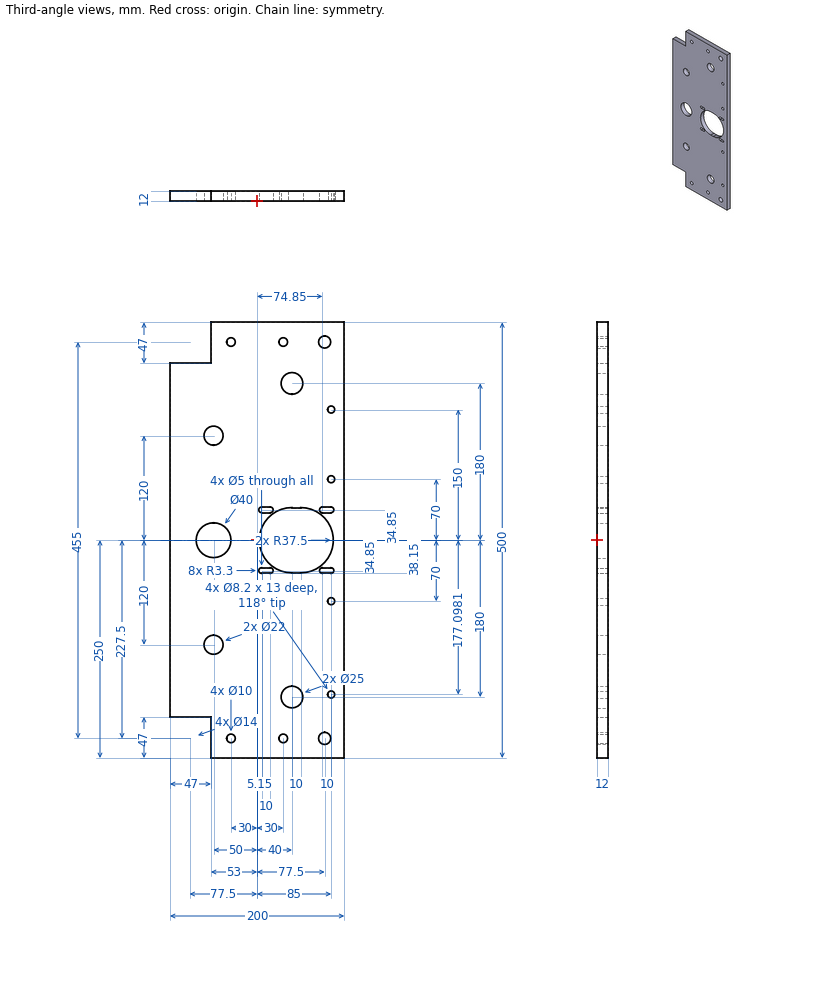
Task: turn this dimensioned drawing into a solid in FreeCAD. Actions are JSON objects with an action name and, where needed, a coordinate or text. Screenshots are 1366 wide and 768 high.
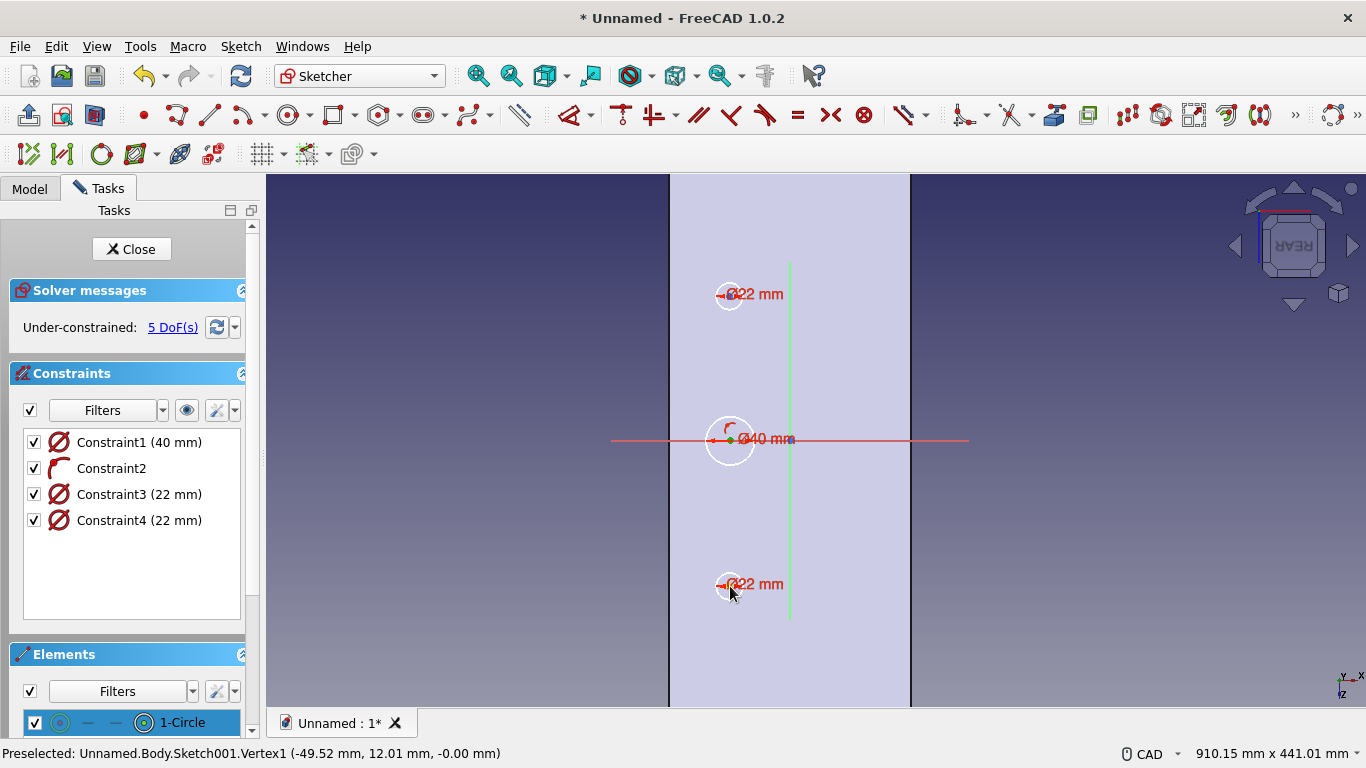
{"action": "left_click", "coordinate": [730, 296]}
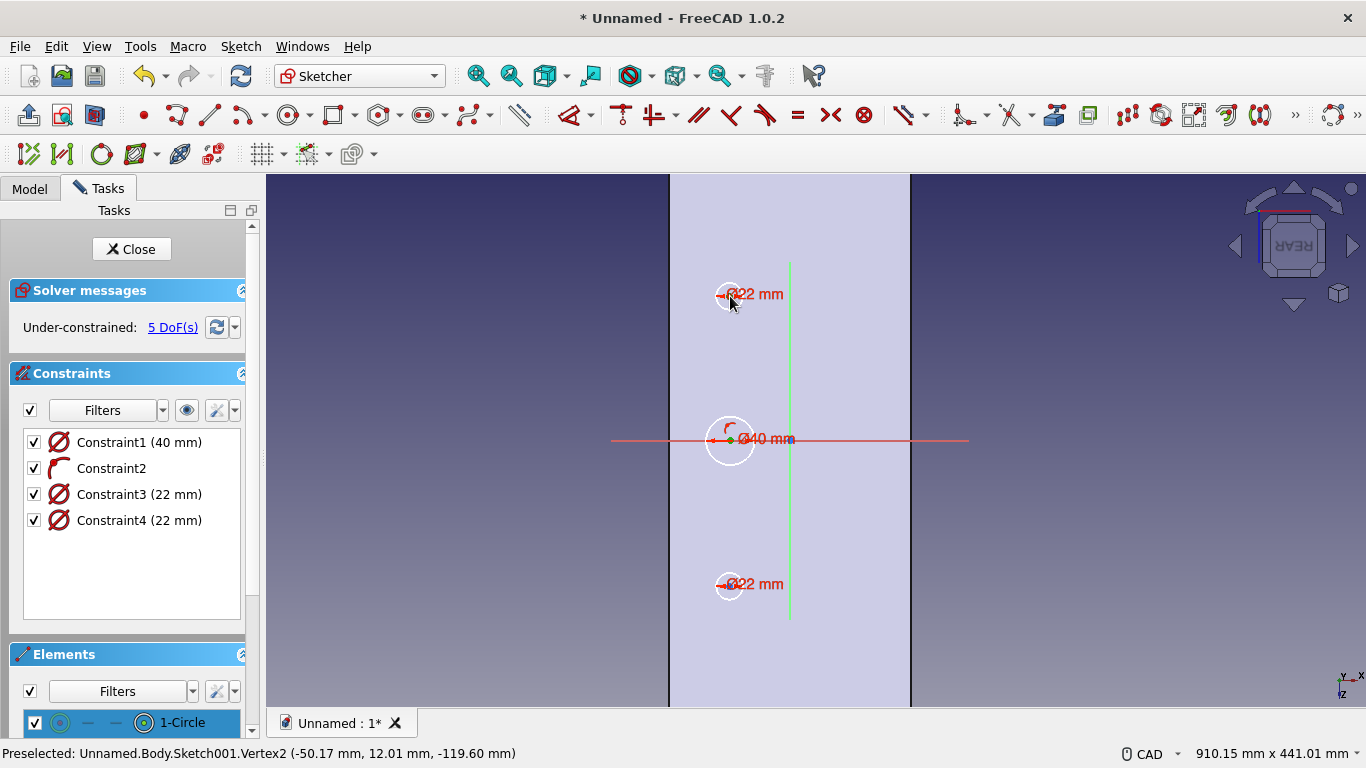
{"action": "key", "text": "v"}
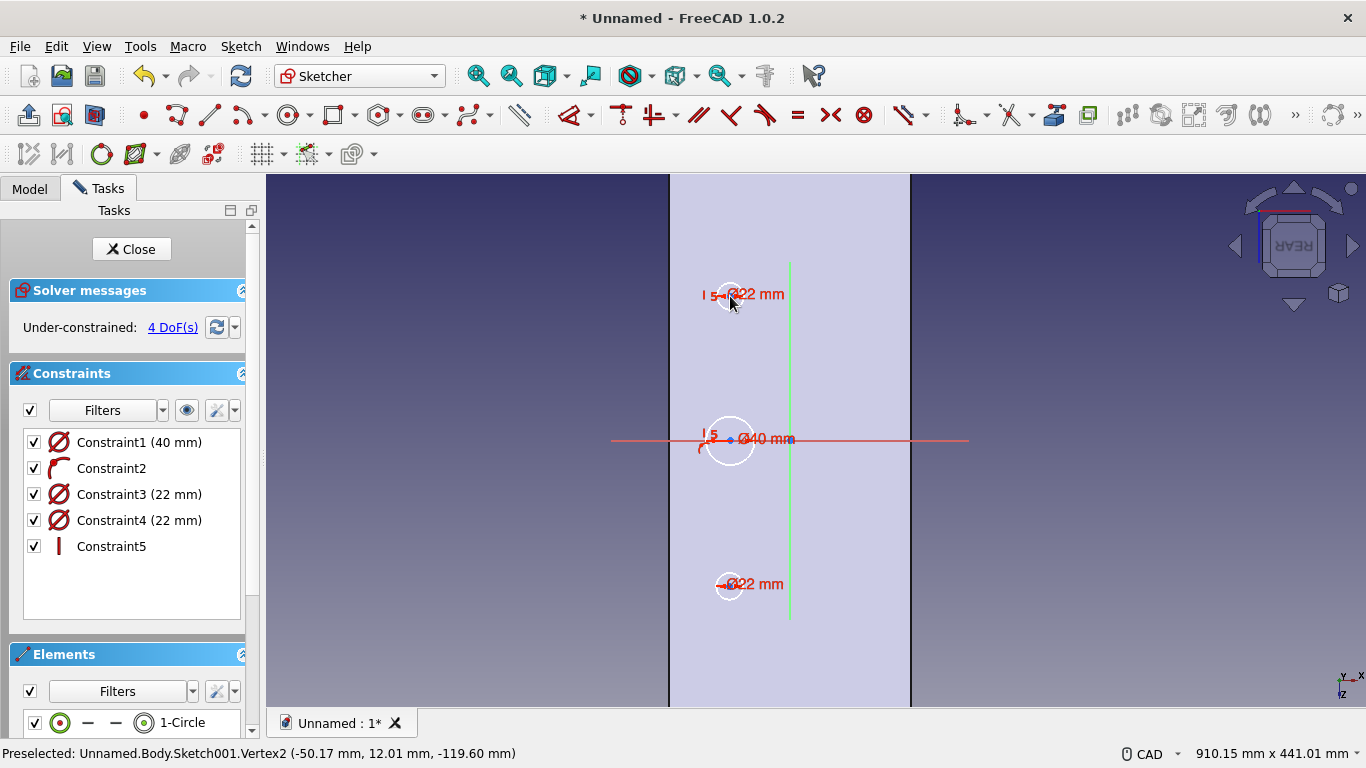
{"action": "left_click", "coordinate": [730, 441]}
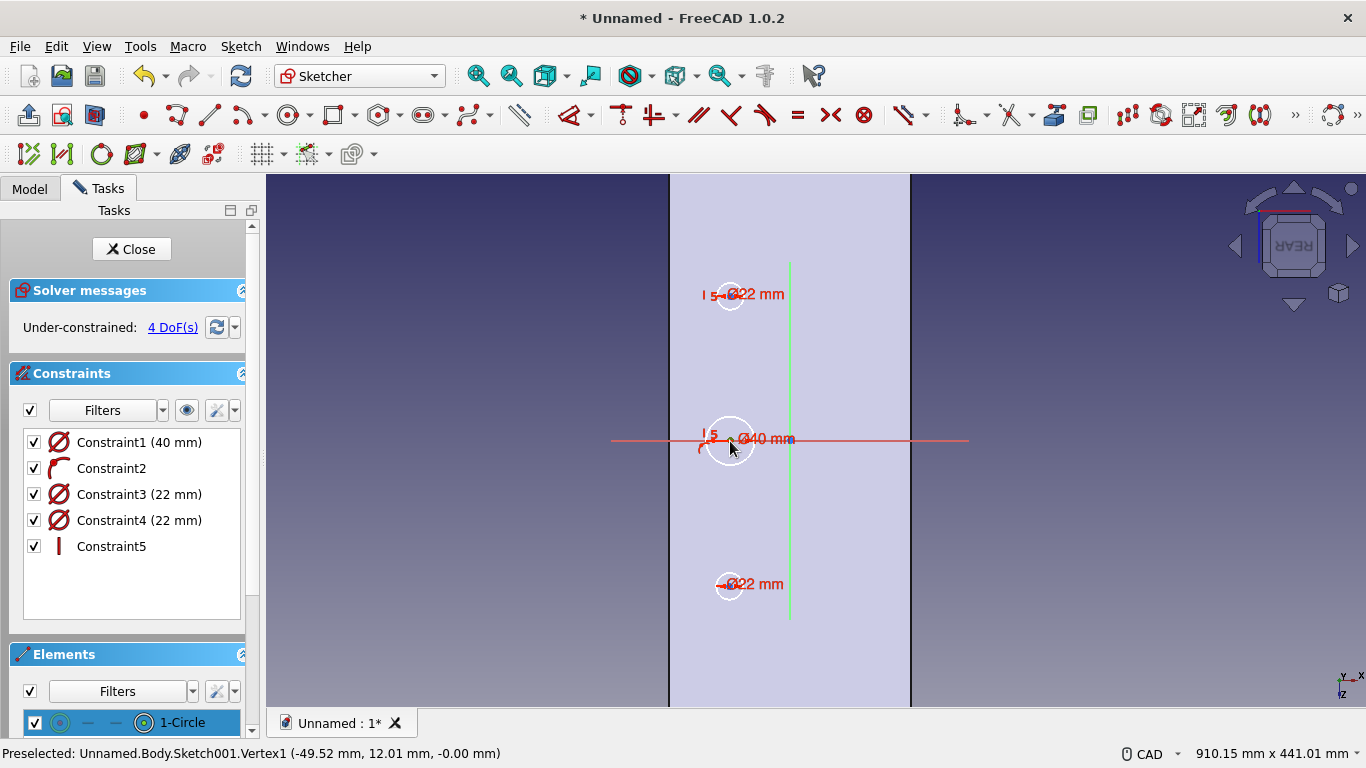
{"action": "left_click", "coordinate": [730, 586]}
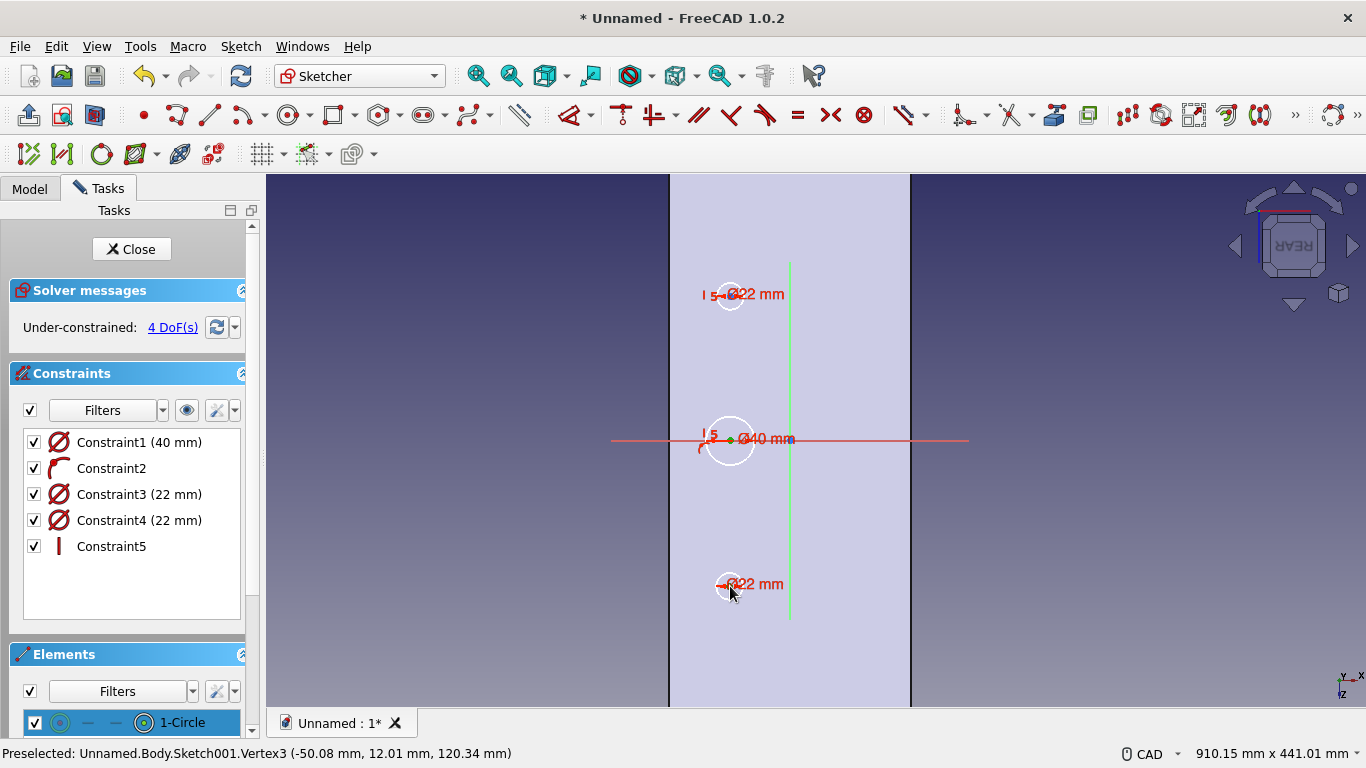
{"action": "key", "text": "v"}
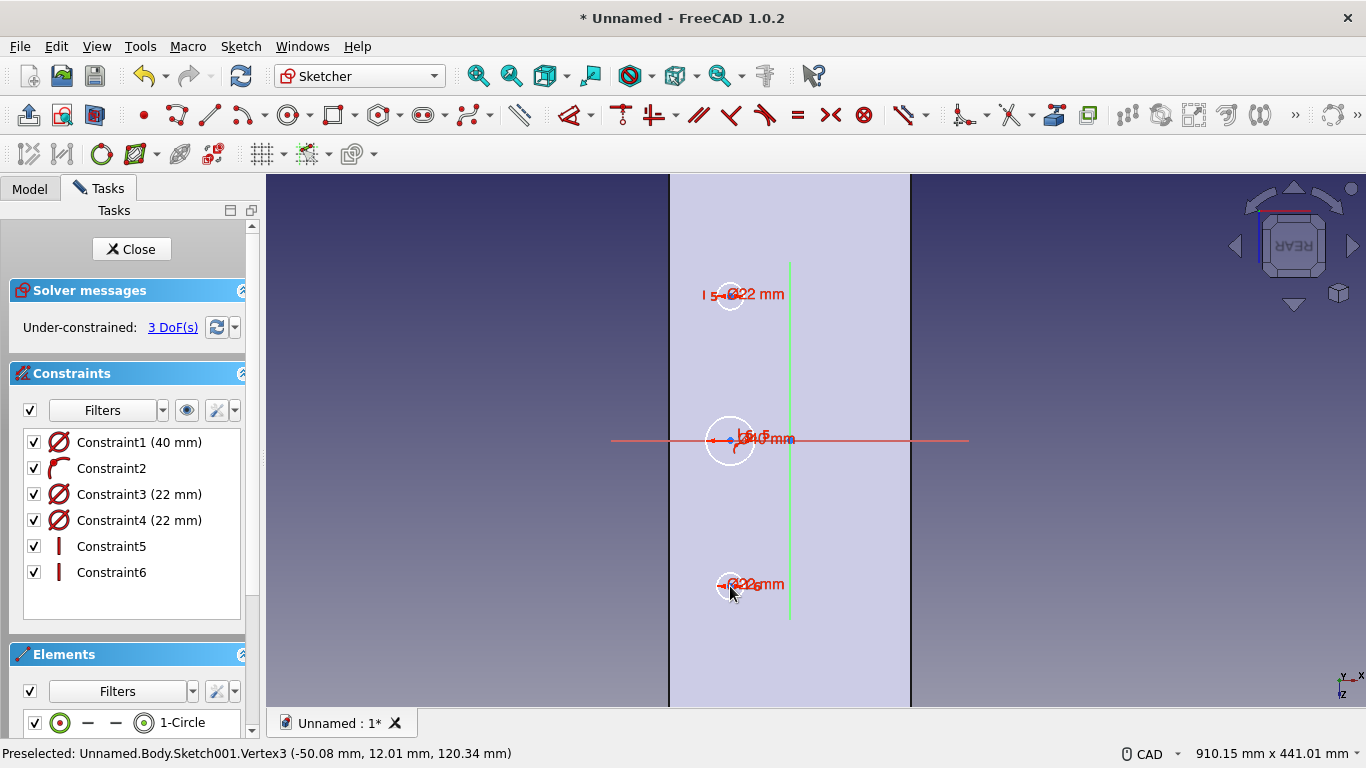
{"action": "key", "text": "d"}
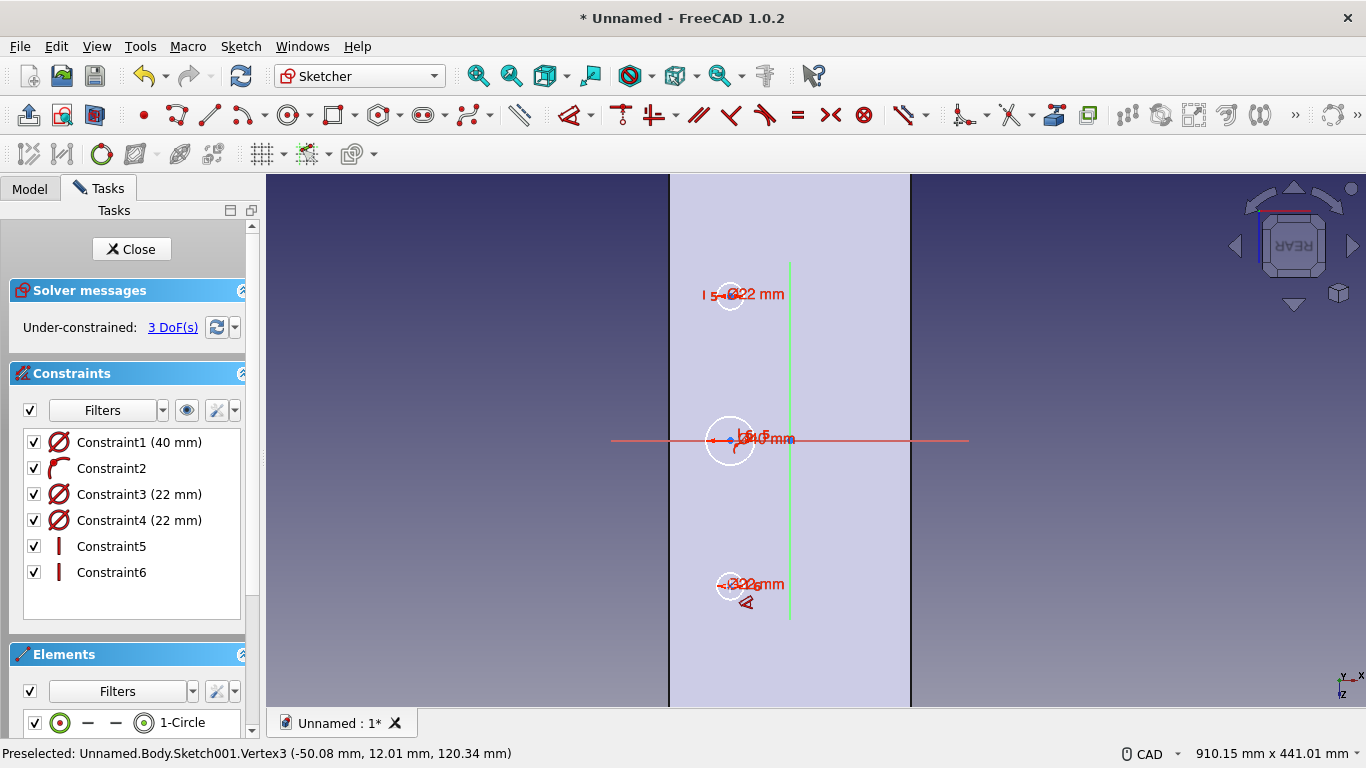
{"action": "left_click", "coordinate": [730, 441]}
{"action": "left_click", "coordinate": [760, 475]}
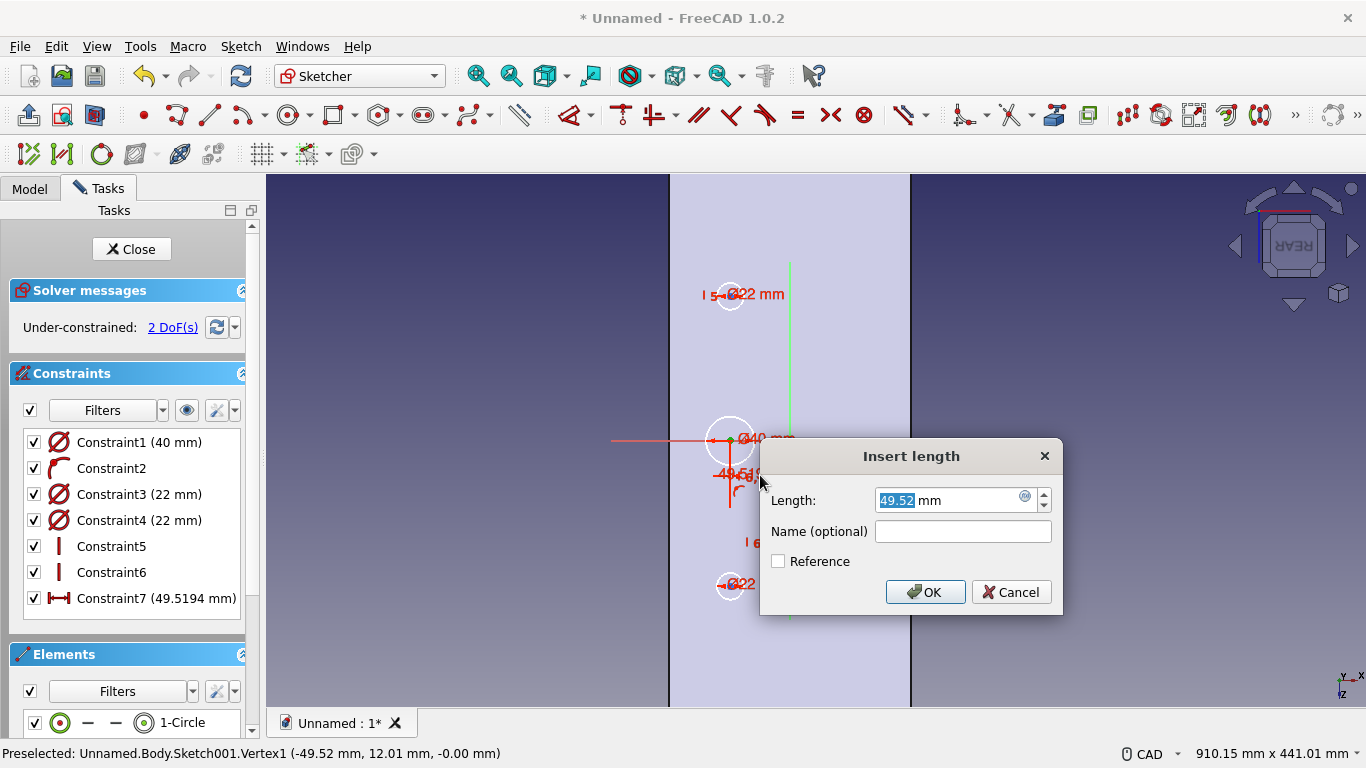
{"action": "type", "text": "50"}
{"action": "key", "text": "Return"}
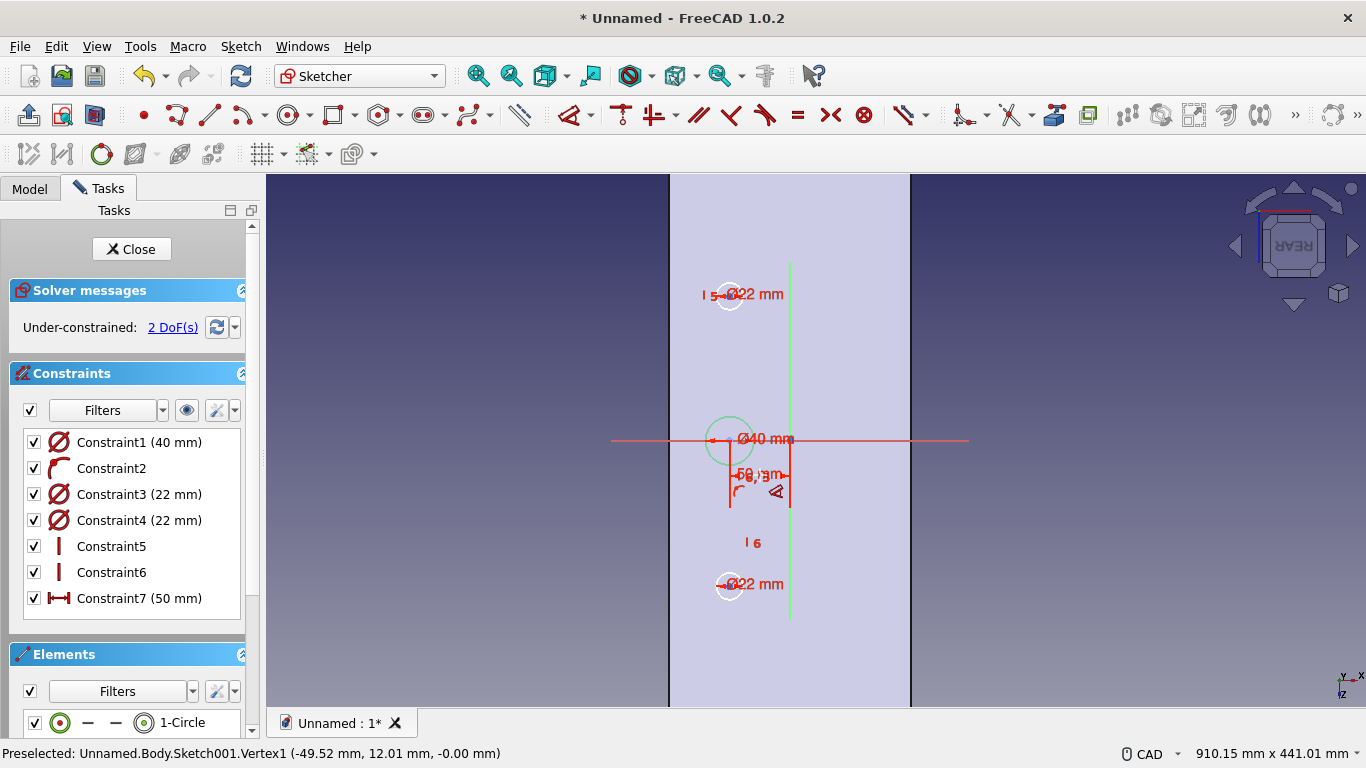
{"action": "left_click", "coordinate": [730, 296]}
{"action": "left_click", "coordinate": [824, 369]}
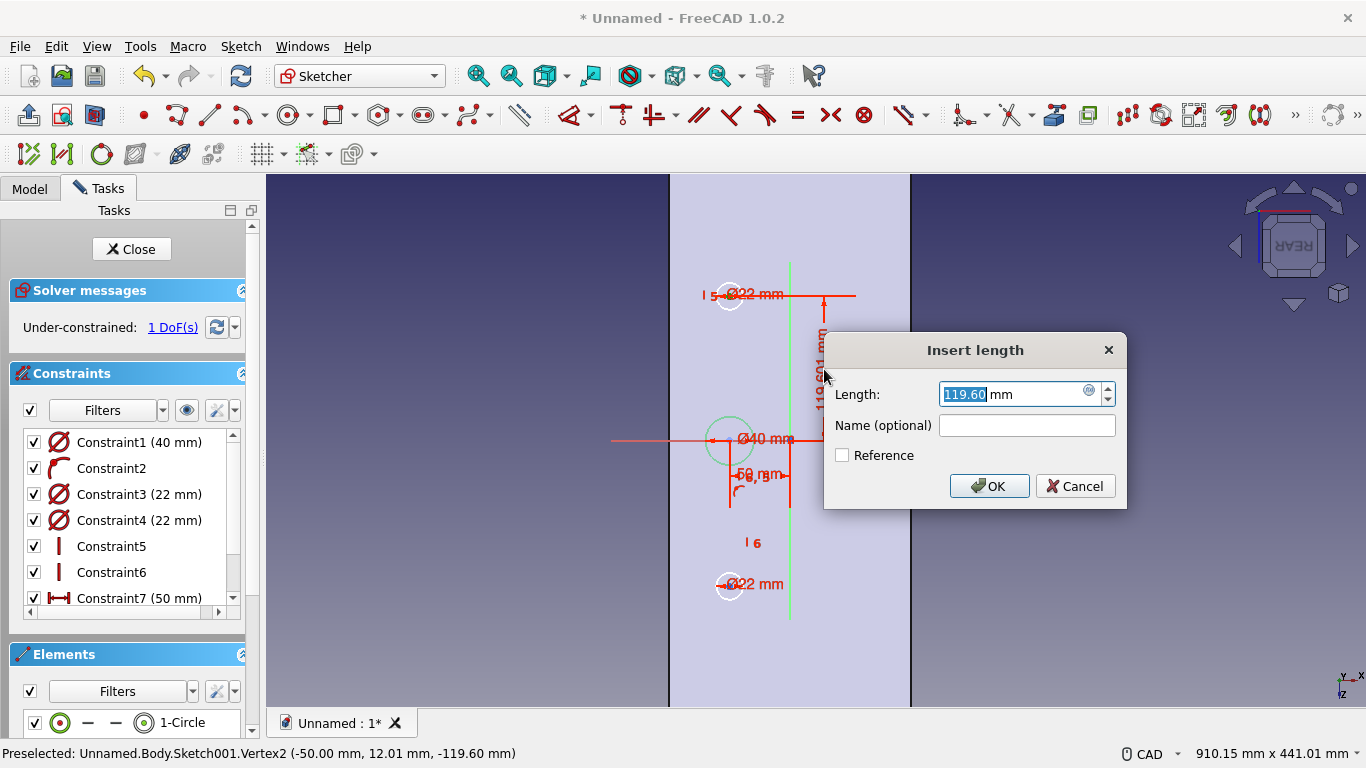
{"action": "type", "text": "120"}
{"action": "key", "text": "Return"}